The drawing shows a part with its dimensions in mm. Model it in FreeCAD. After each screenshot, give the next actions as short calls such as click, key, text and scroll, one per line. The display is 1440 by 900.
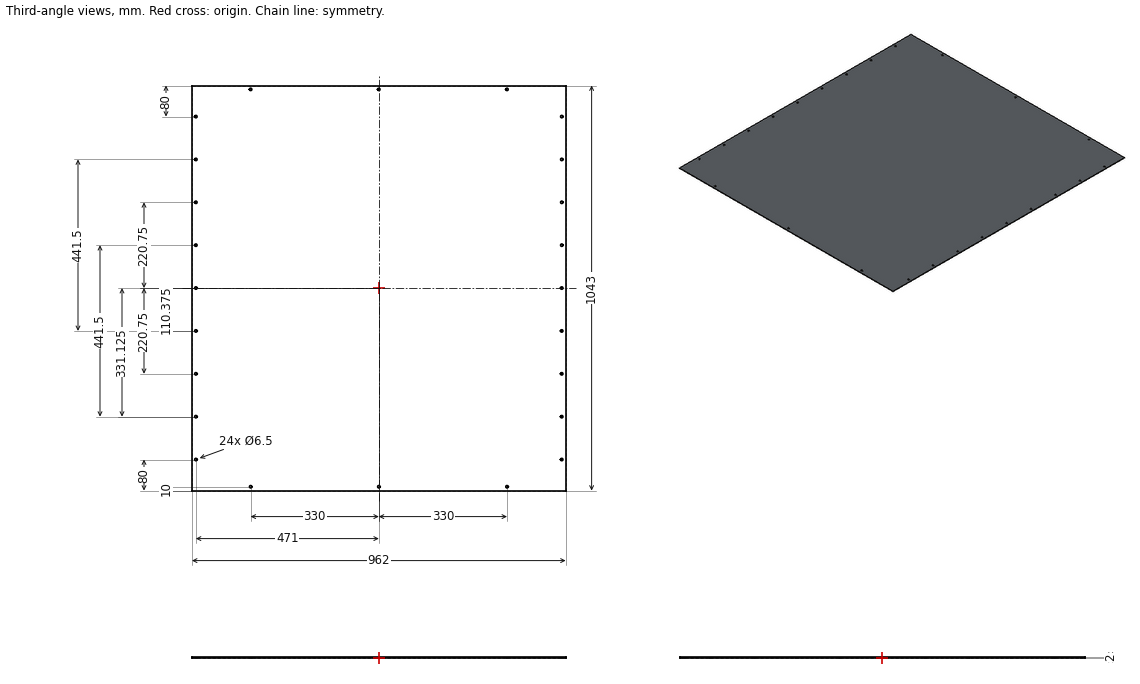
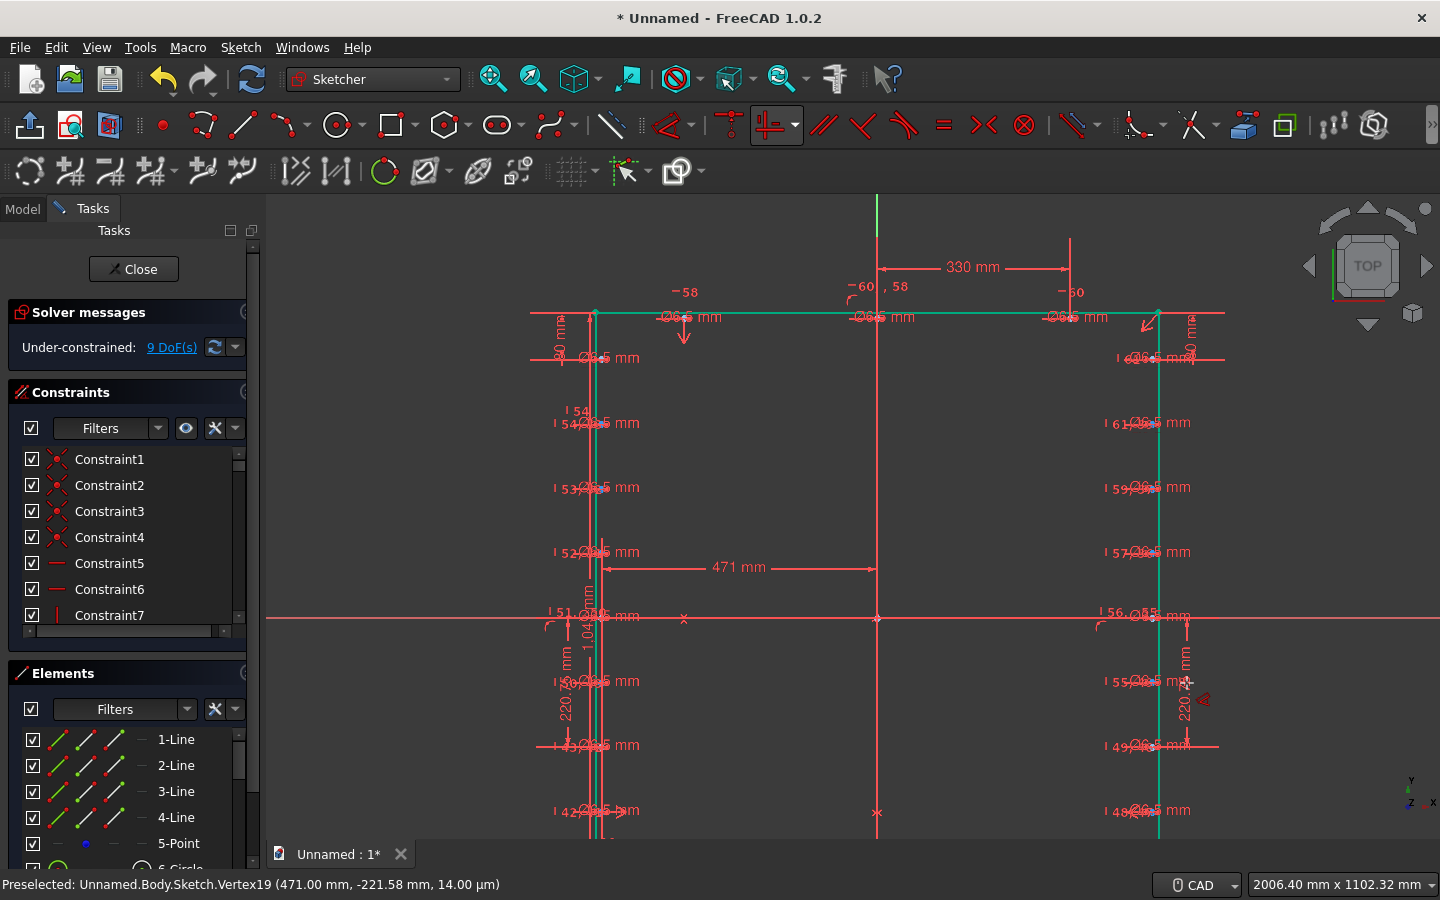
click(602, 489)
click(568, 554)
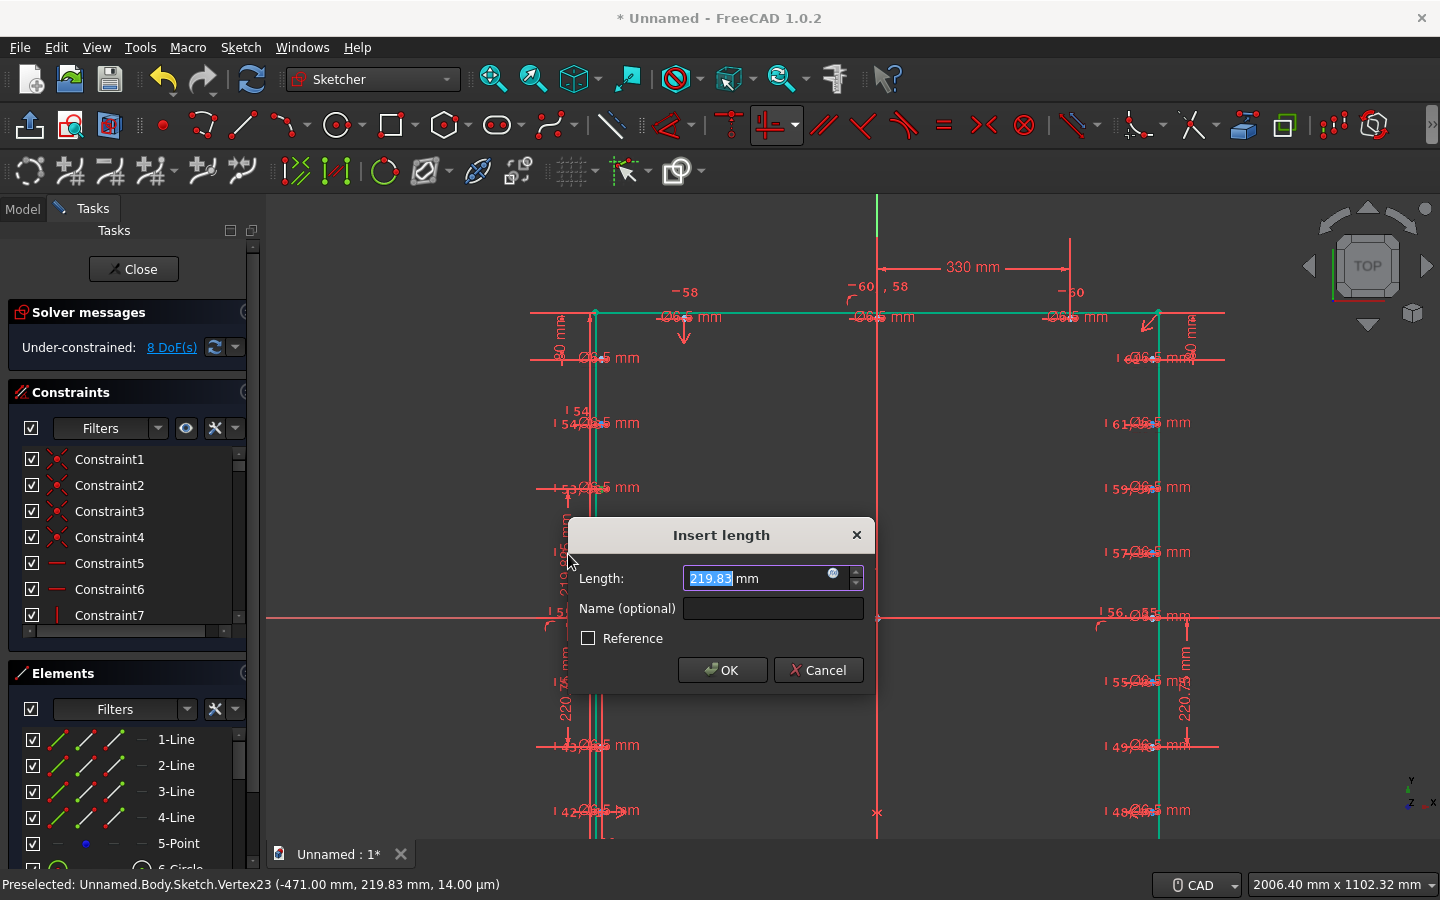
text(220.75)
key(Return)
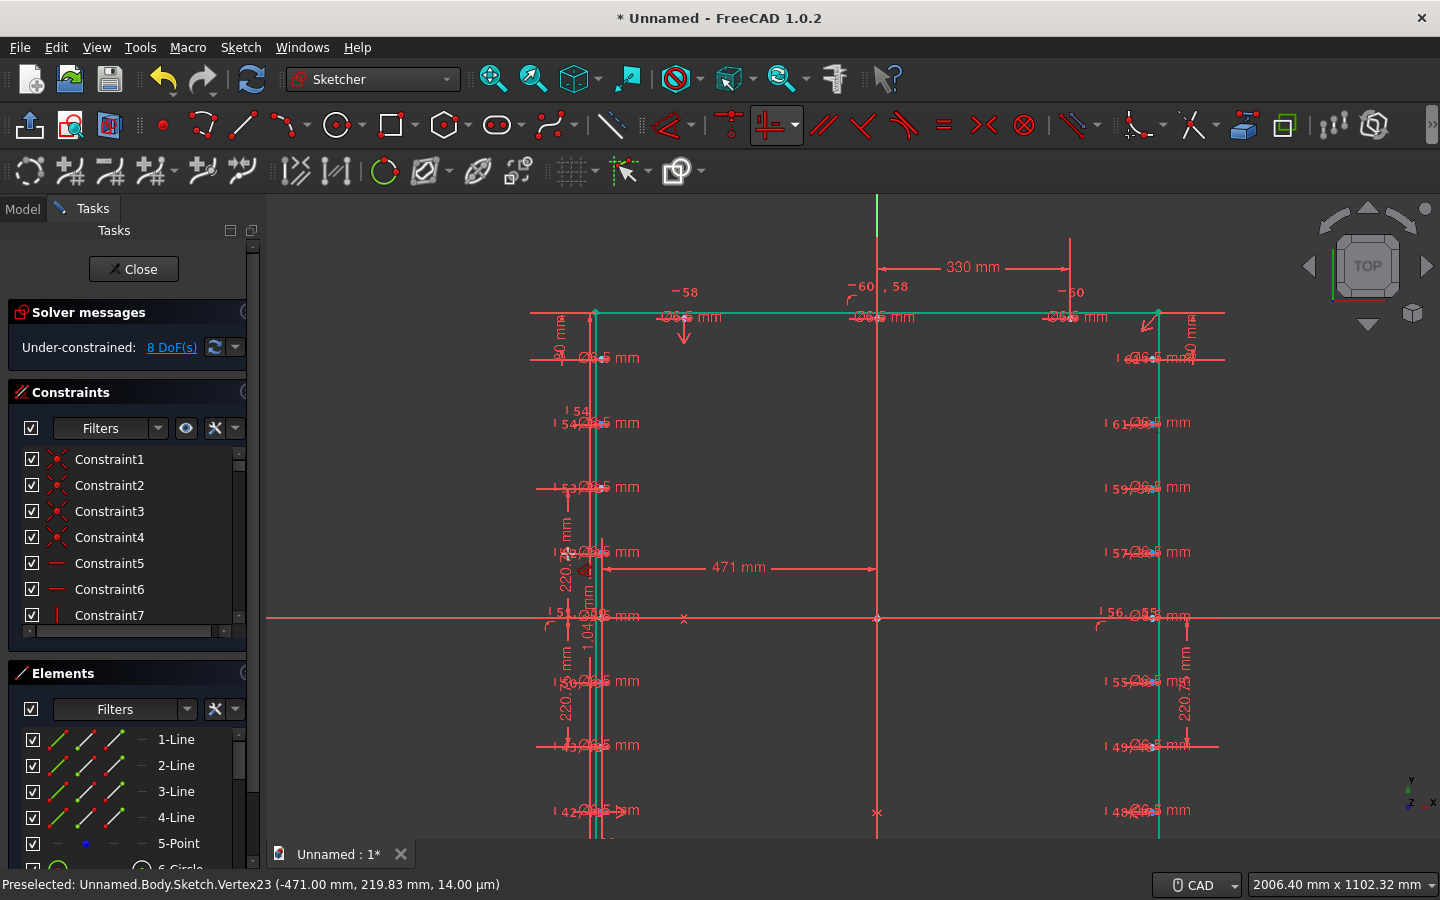
click(1153, 489)
click(1187, 554)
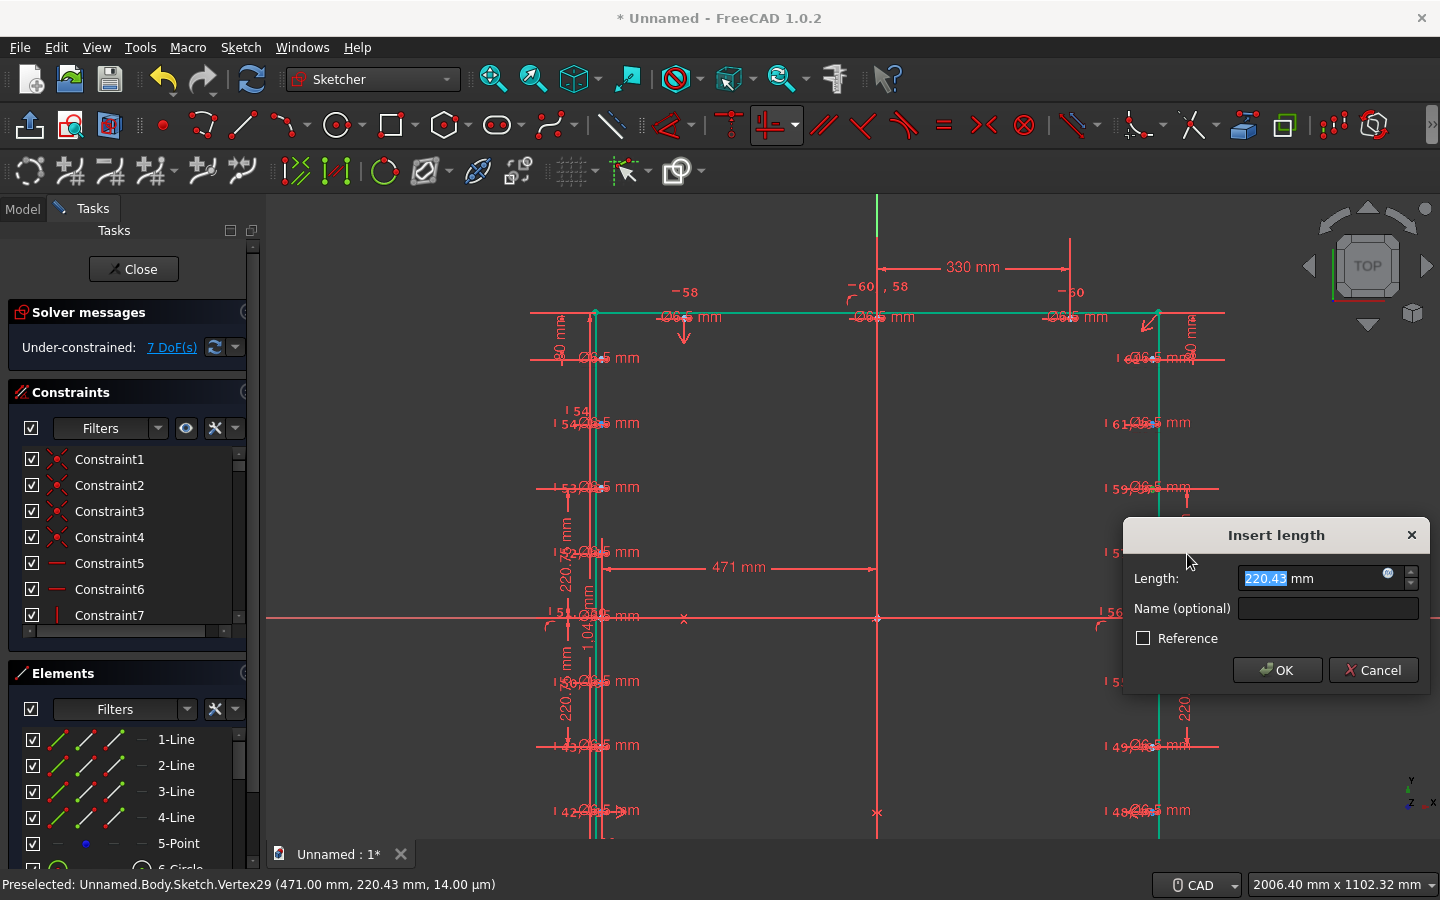
text(220.75)
key(Return)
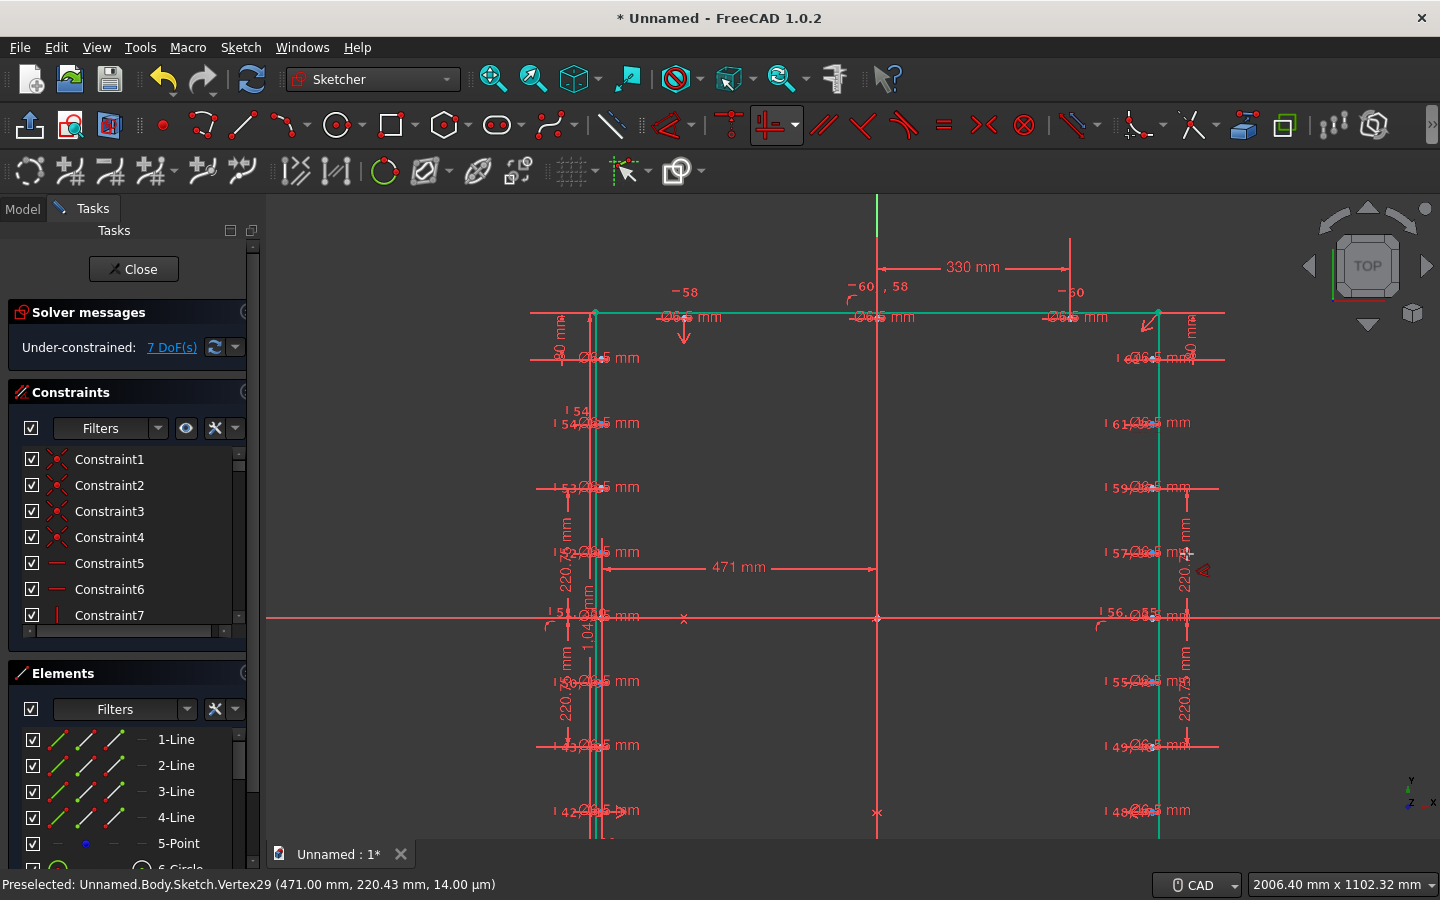
scroll(596, 310, down, 2)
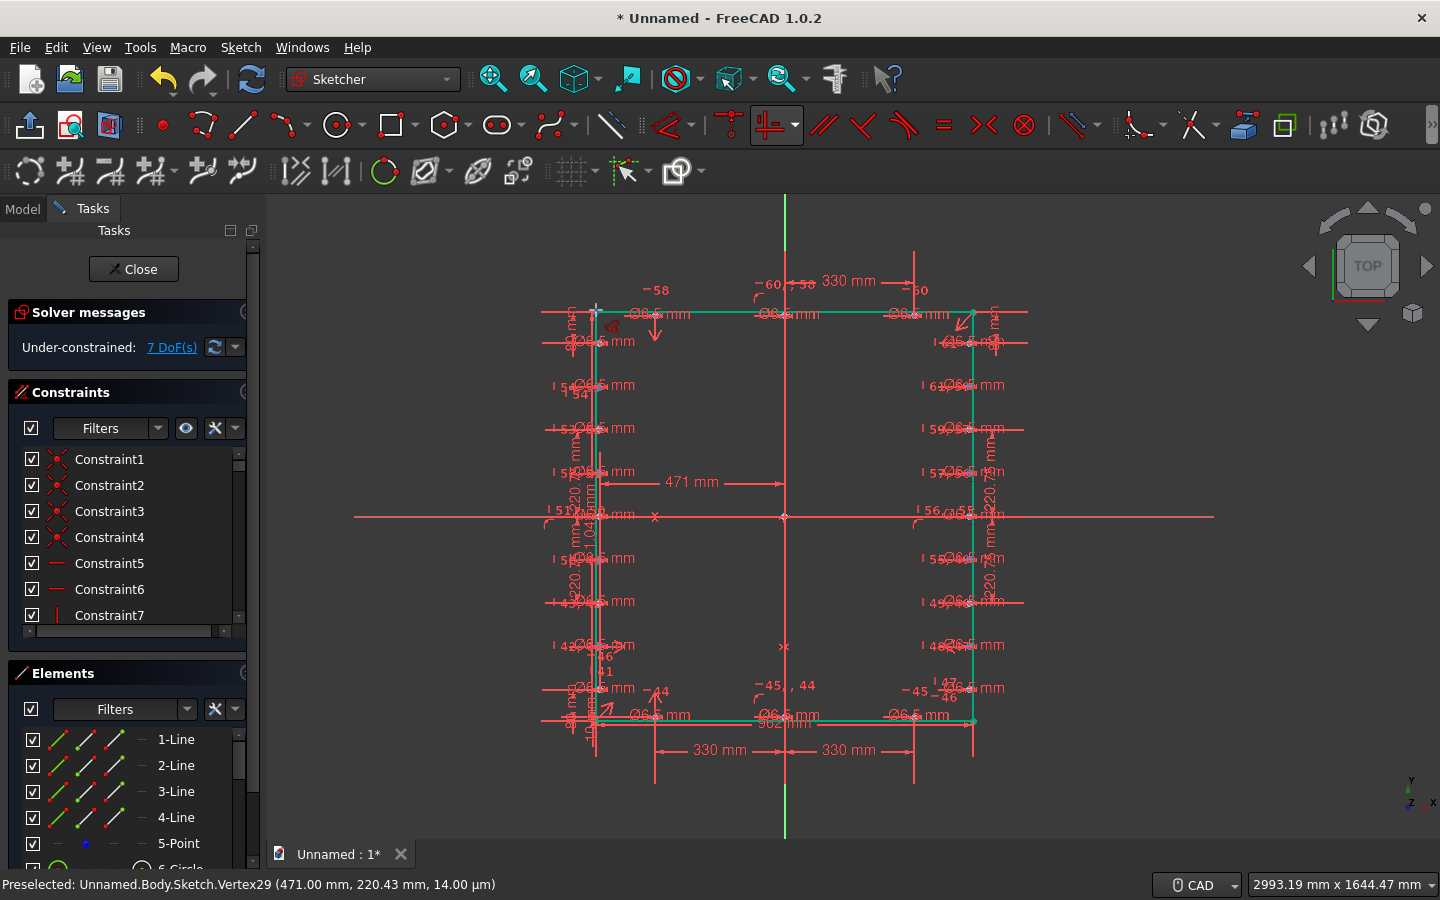
click(600, 647)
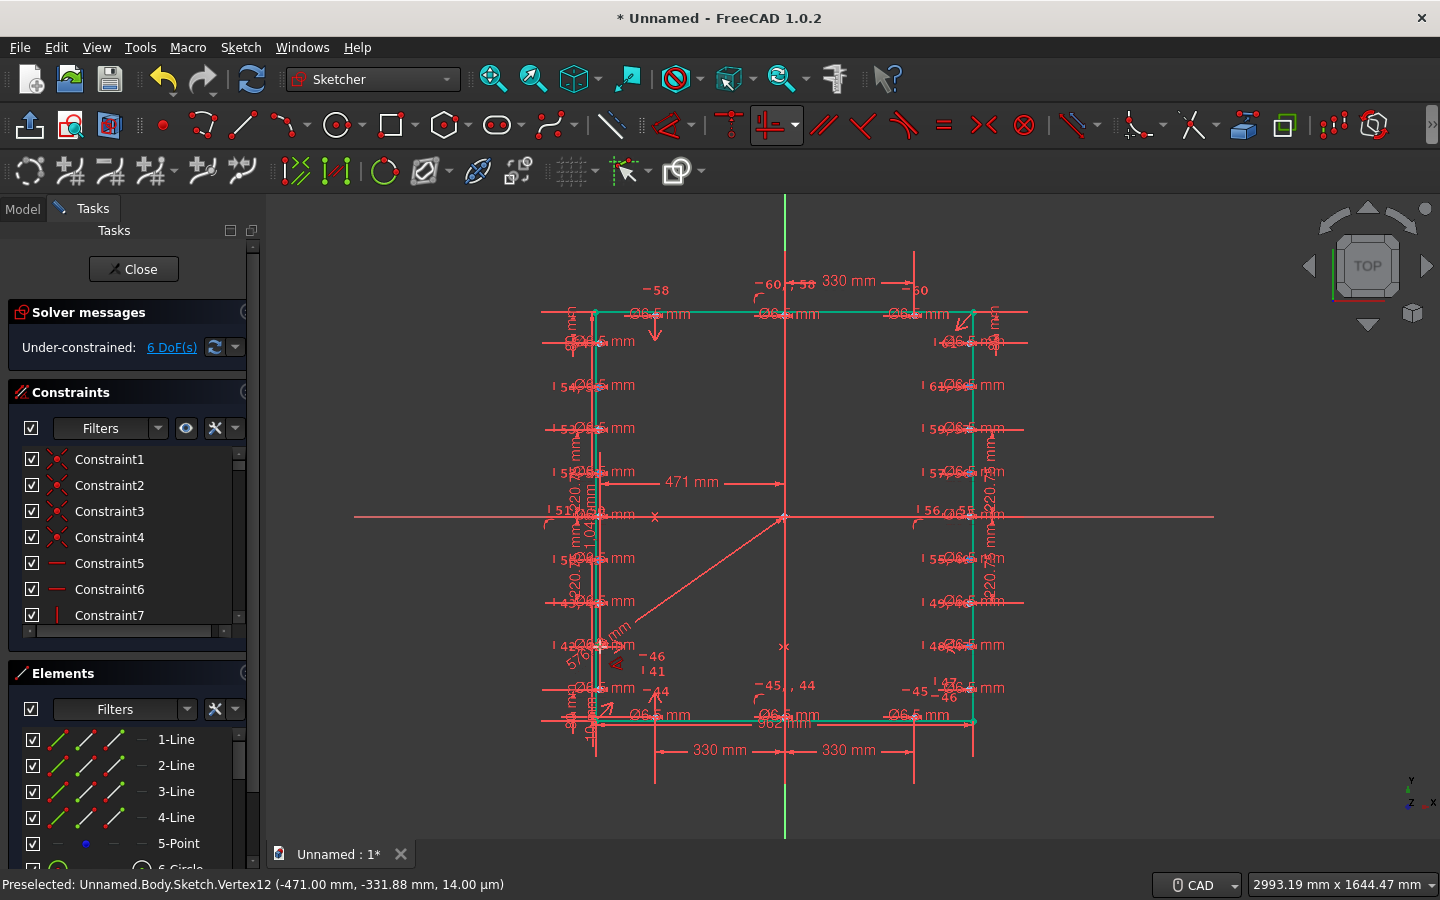
click(600, 474)
click(566, 600)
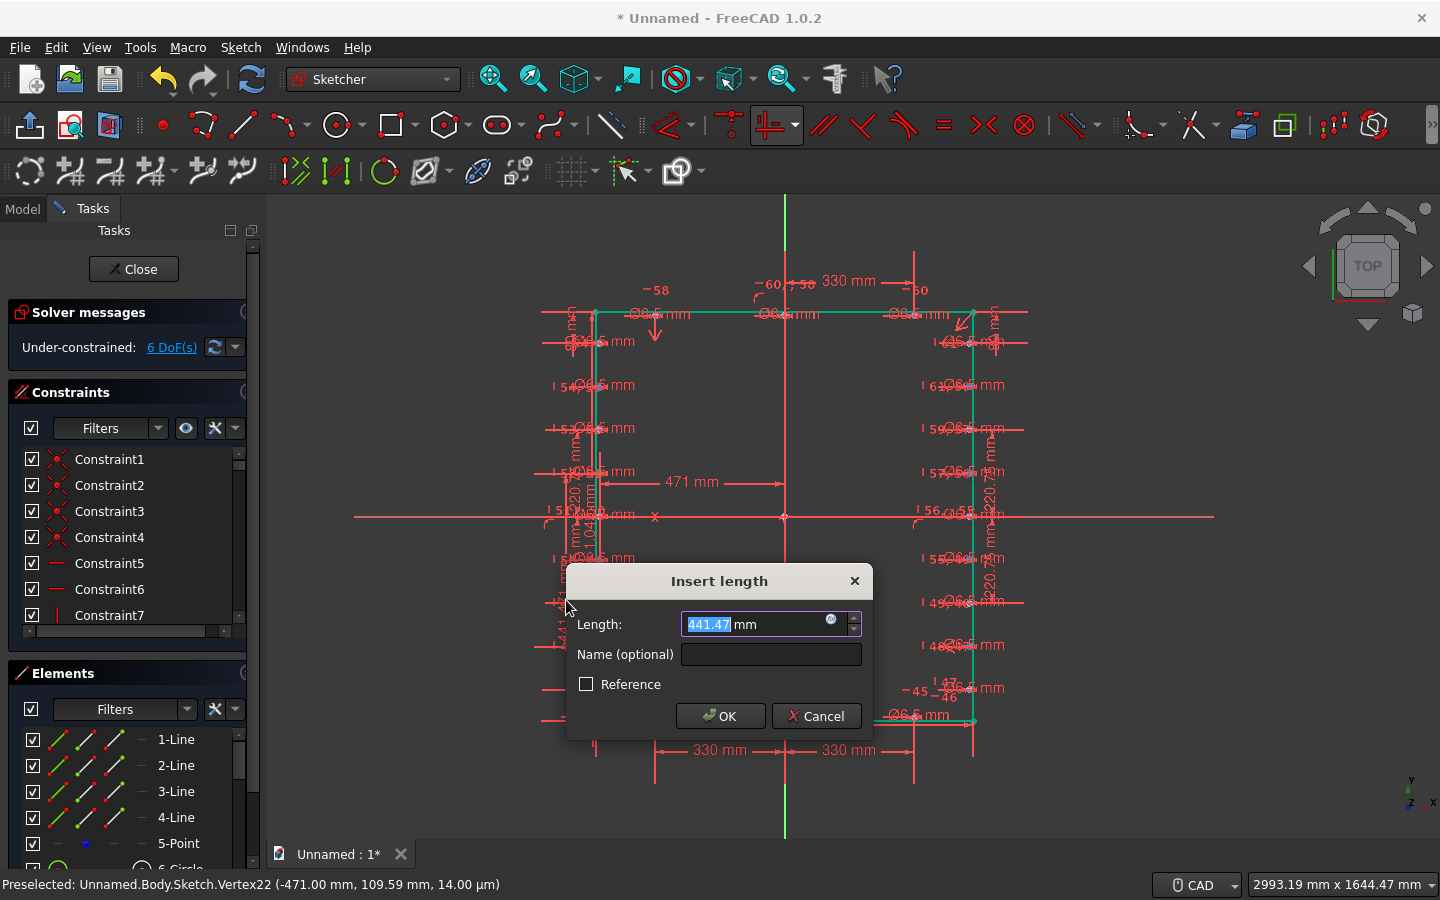
text(441.5)
key(Return)